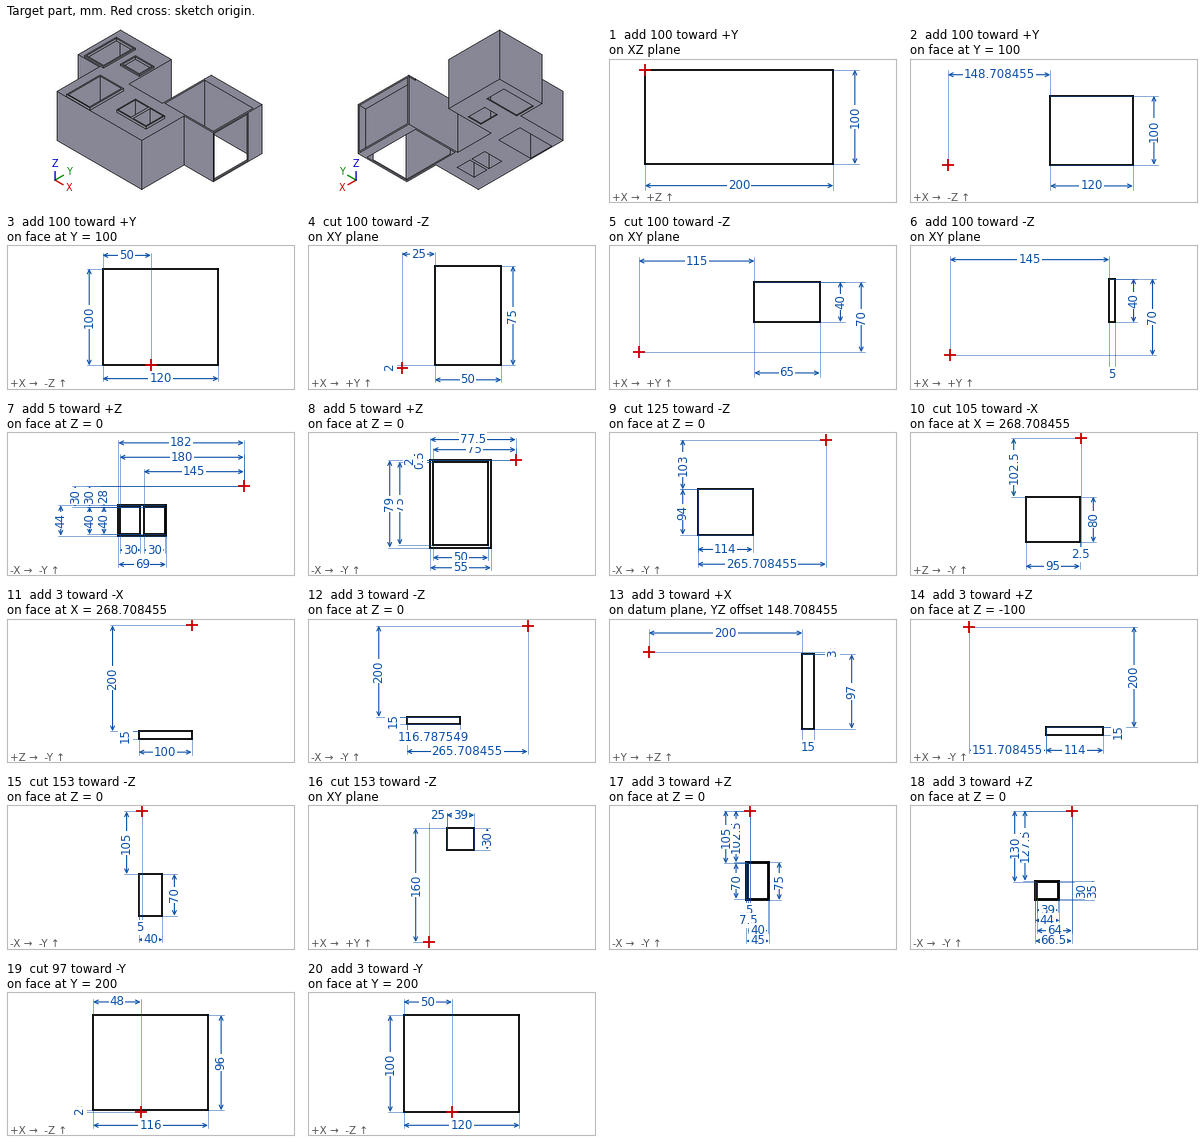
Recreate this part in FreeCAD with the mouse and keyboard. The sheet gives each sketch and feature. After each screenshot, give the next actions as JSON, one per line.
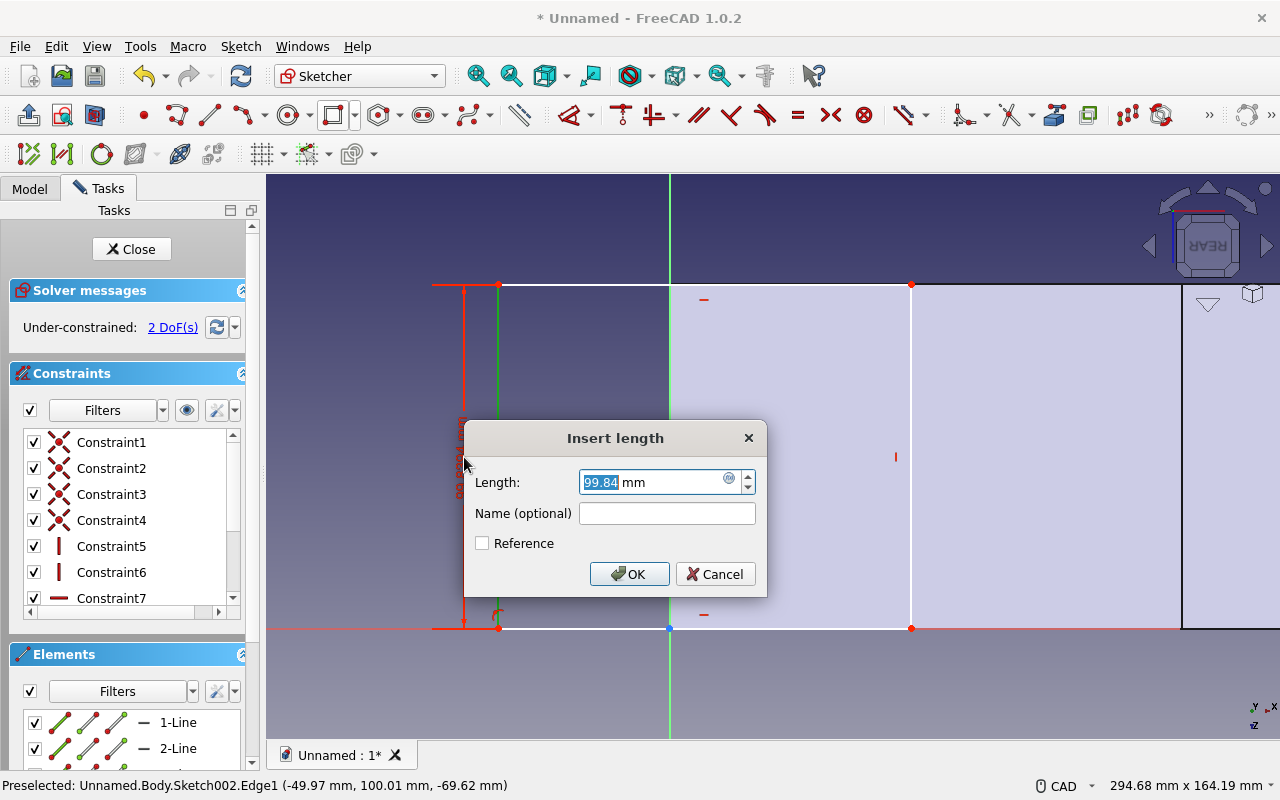
{"action": "type", "text": "100"}
{"action": "key", "text": "Return"}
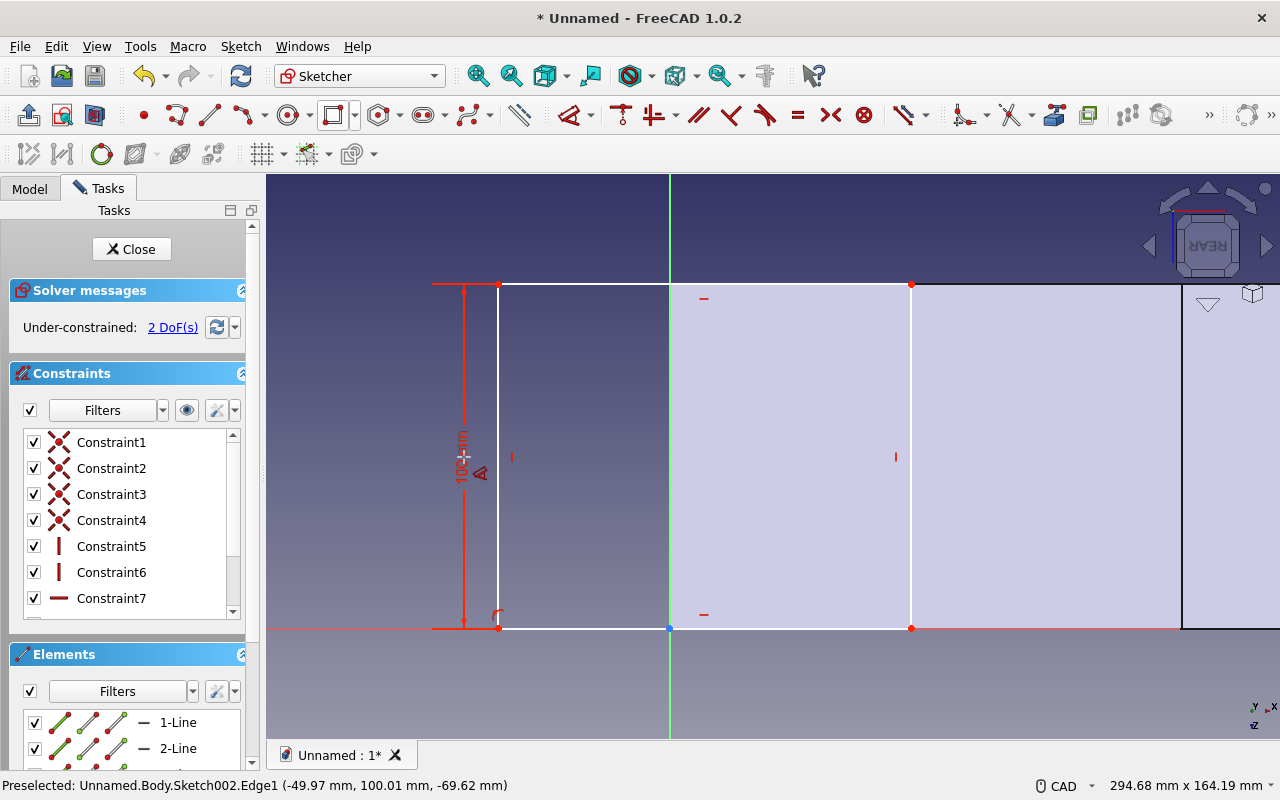
{"action": "left_click", "coordinate": [622, 629]}
{"action": "left_click", "coordinate": [705, 663]}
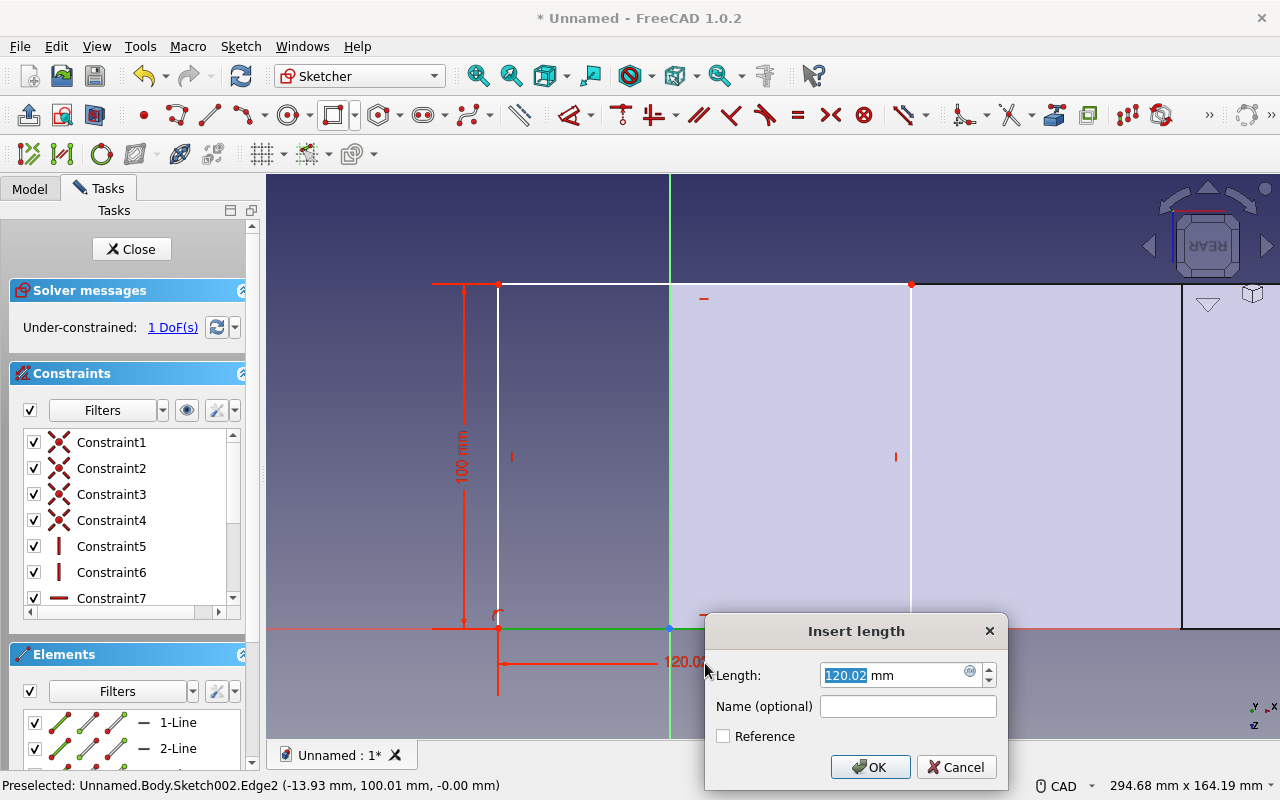
{"action": "type", "text": "120"}
{"action": "key", "text": "Return"}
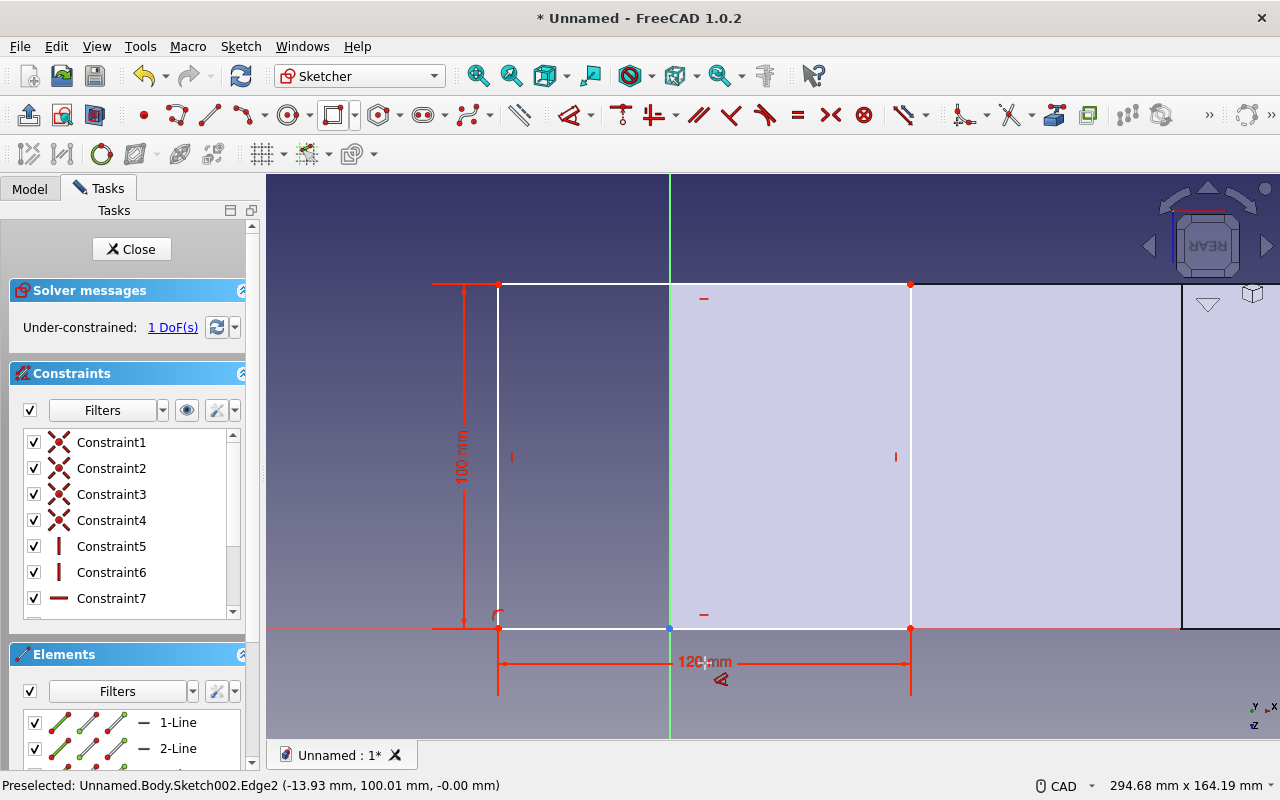
{"action": "left_click", "coordinate": [498, 284]}
{"action": "left_click", "coordinate": [584, 663]}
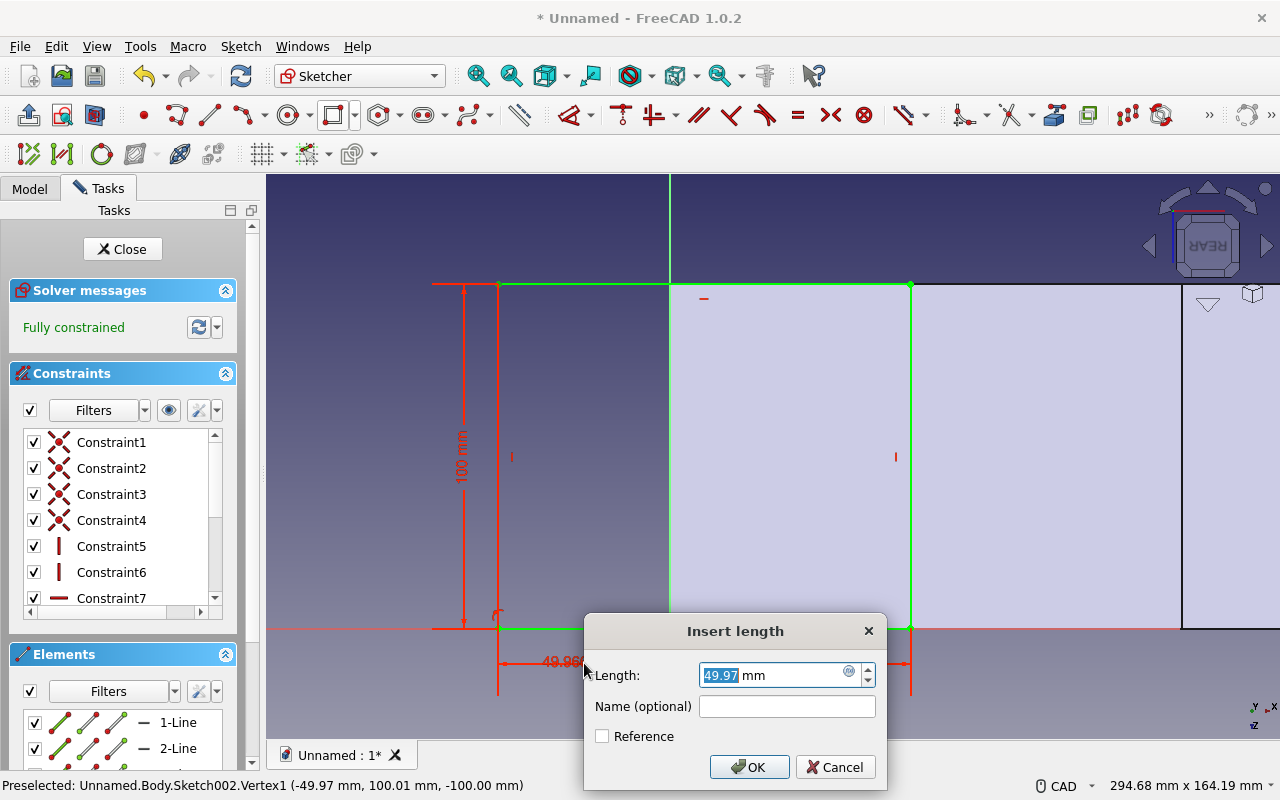
{"action": "type", "text": "50"}
{"action": "key", "text": "Return"}
{"action": "key", "text": "Escape"}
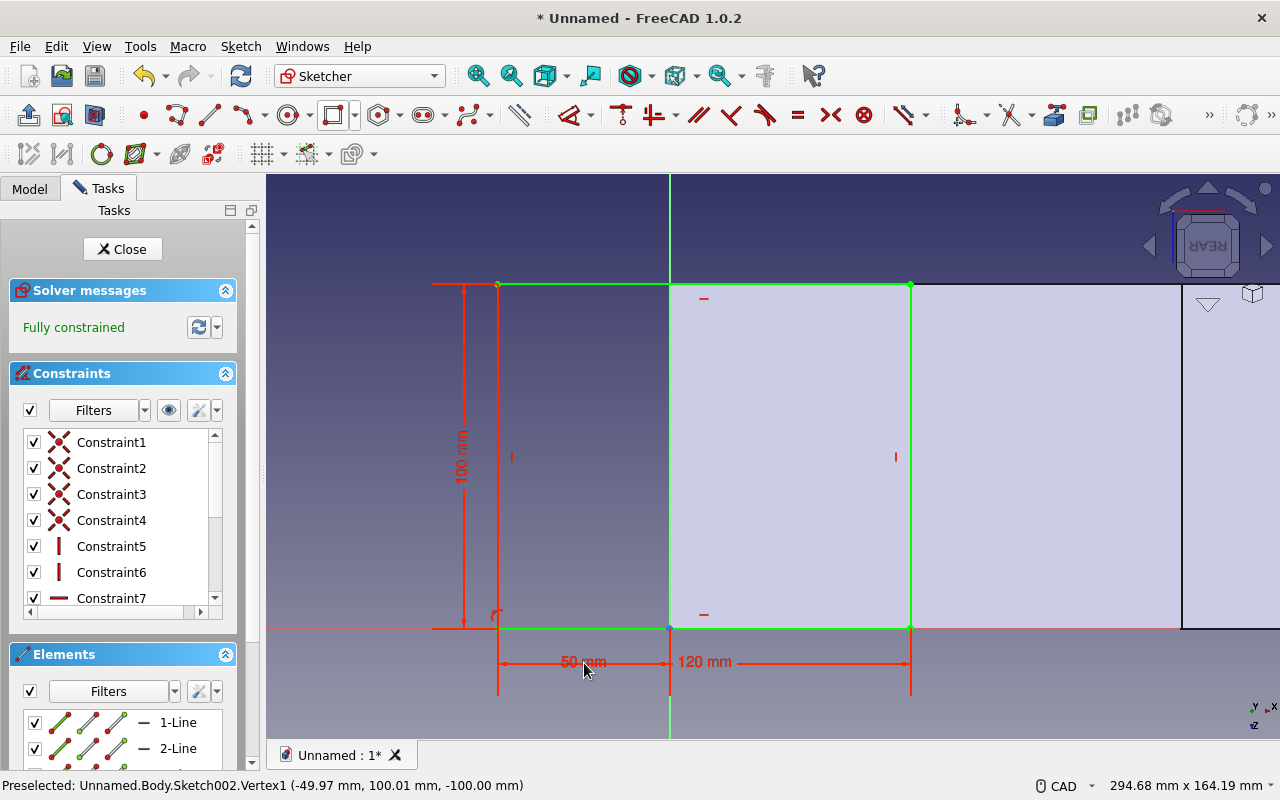
{"action": "left_click", "coordinate": [123, 249]}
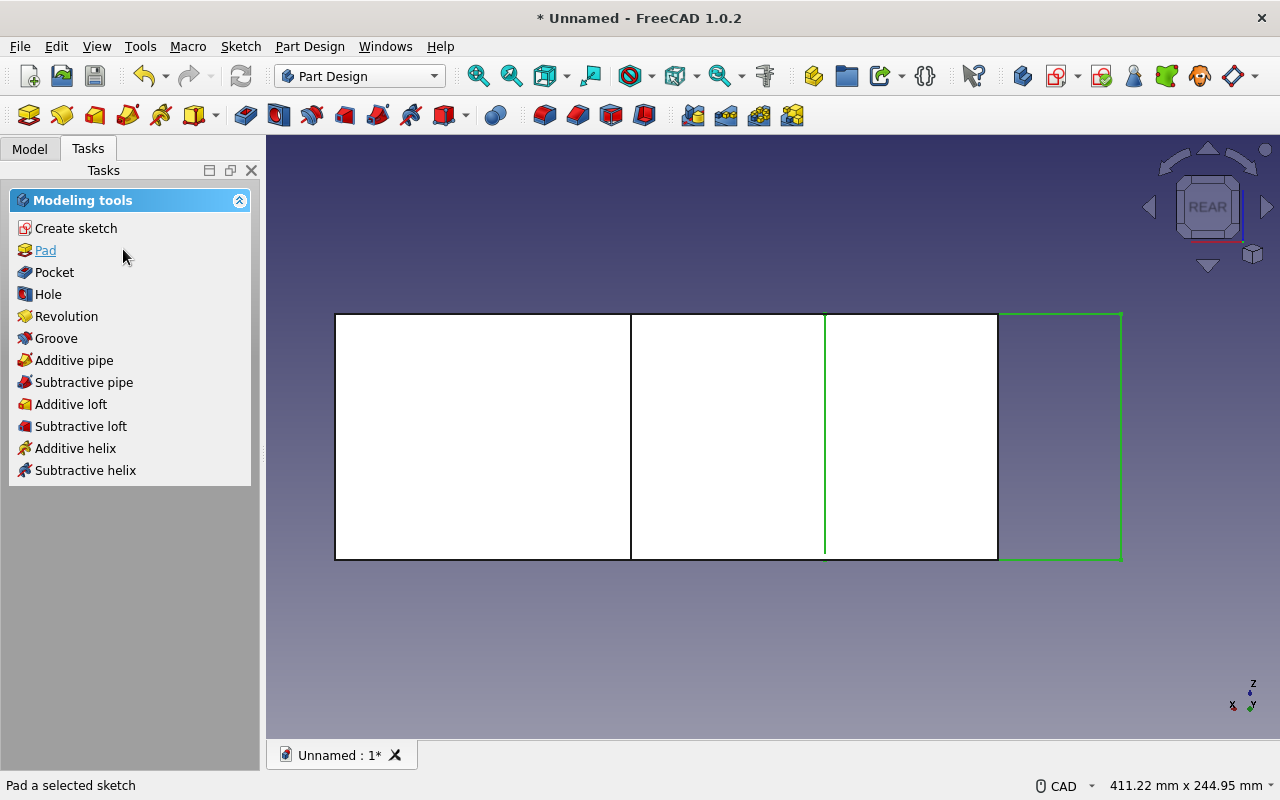
{"action": "left_click", "coordinate": [29, 116]}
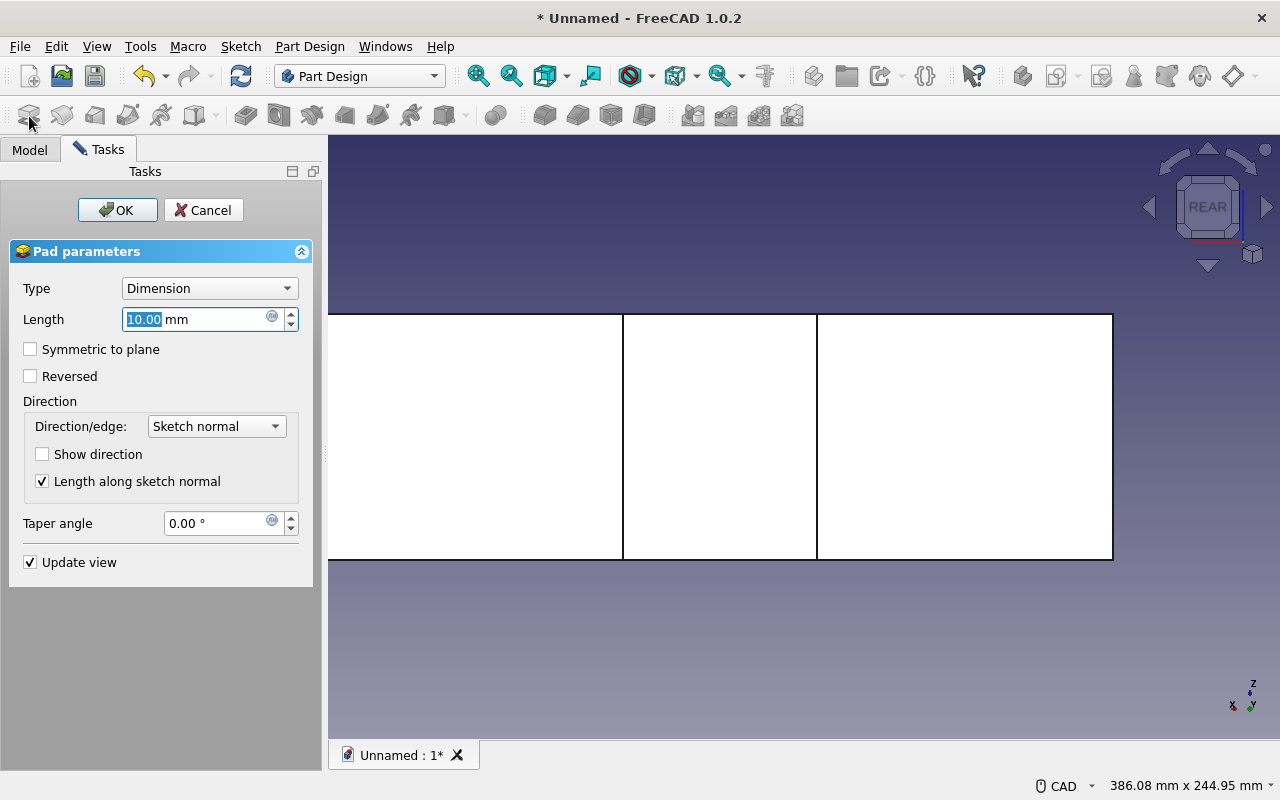
{"action": "type", "text": "100"}
{"action": "key", "text": "Tab"}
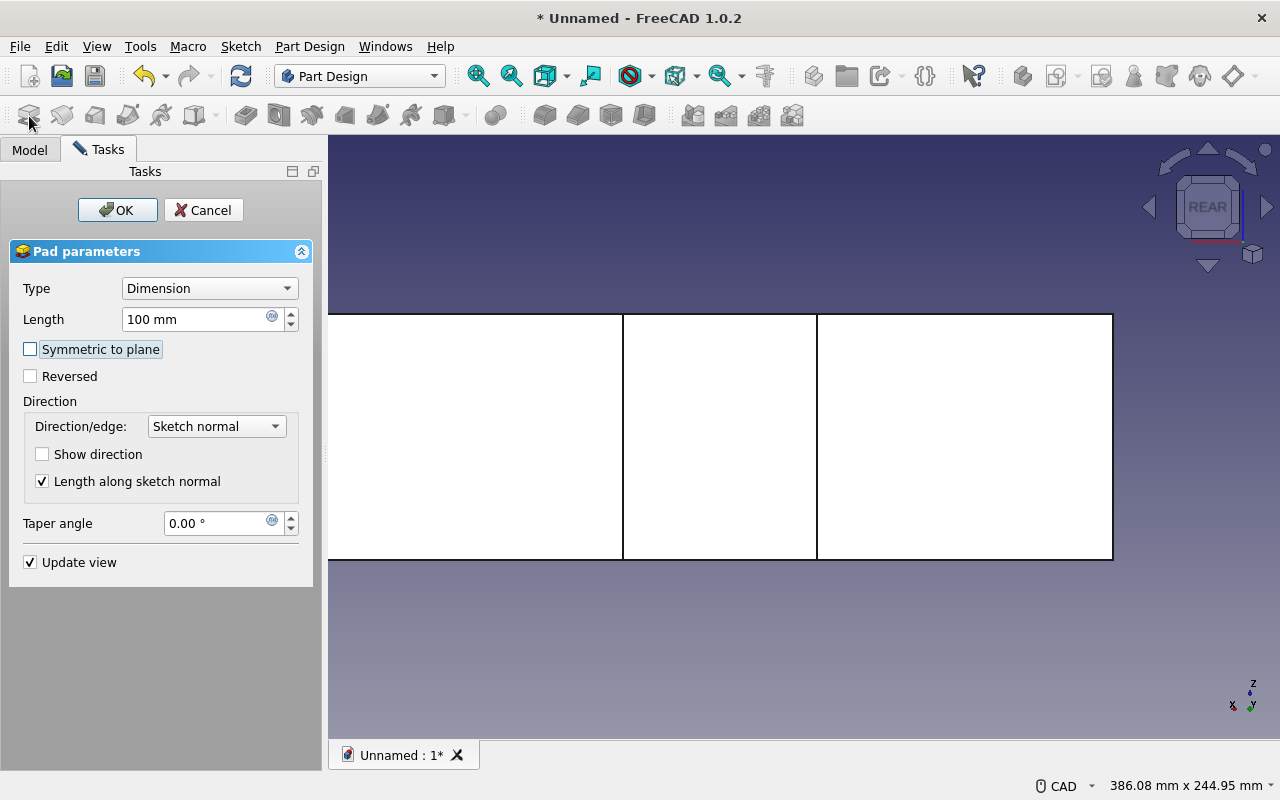
{"action": "left_click", "coordinate": [118, 210]}